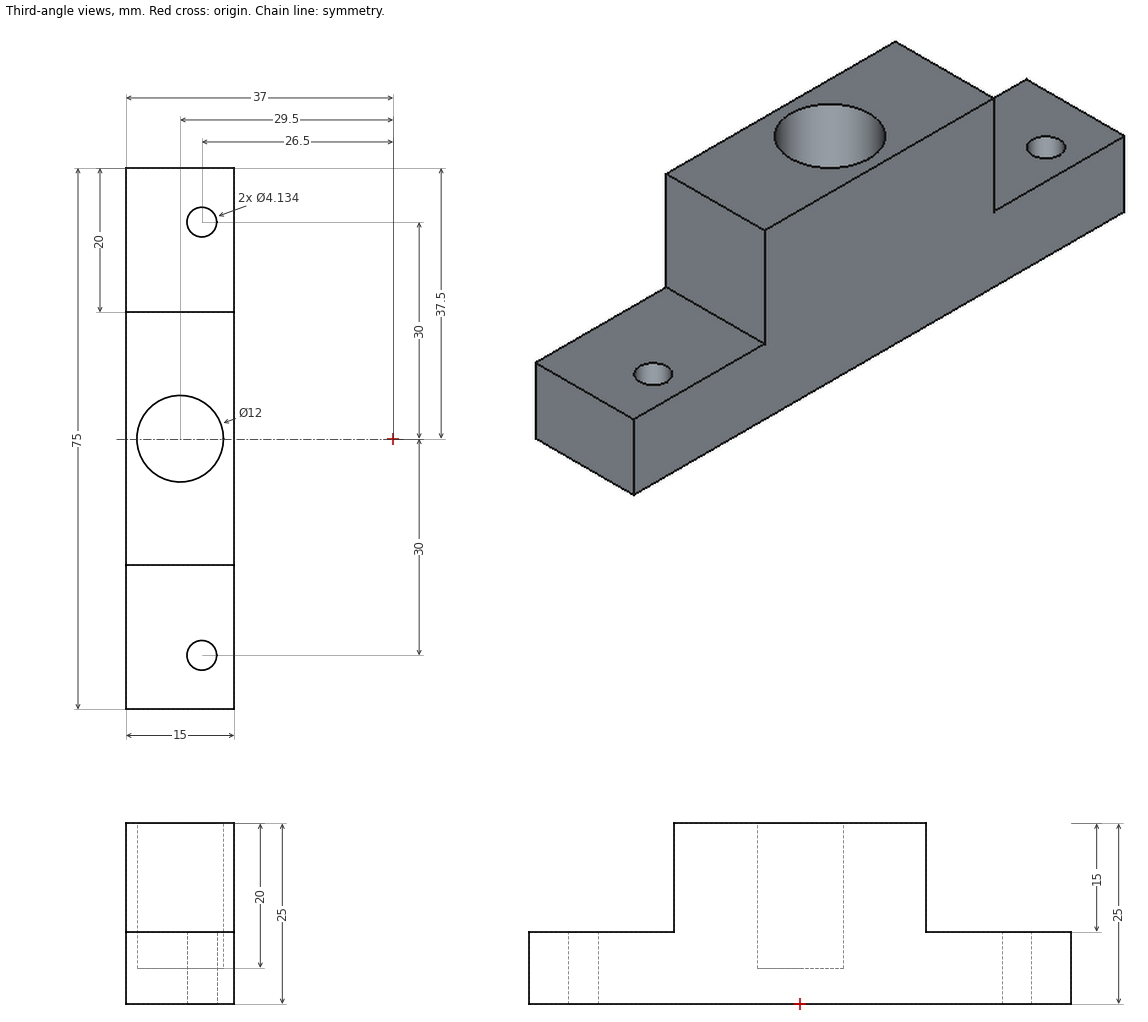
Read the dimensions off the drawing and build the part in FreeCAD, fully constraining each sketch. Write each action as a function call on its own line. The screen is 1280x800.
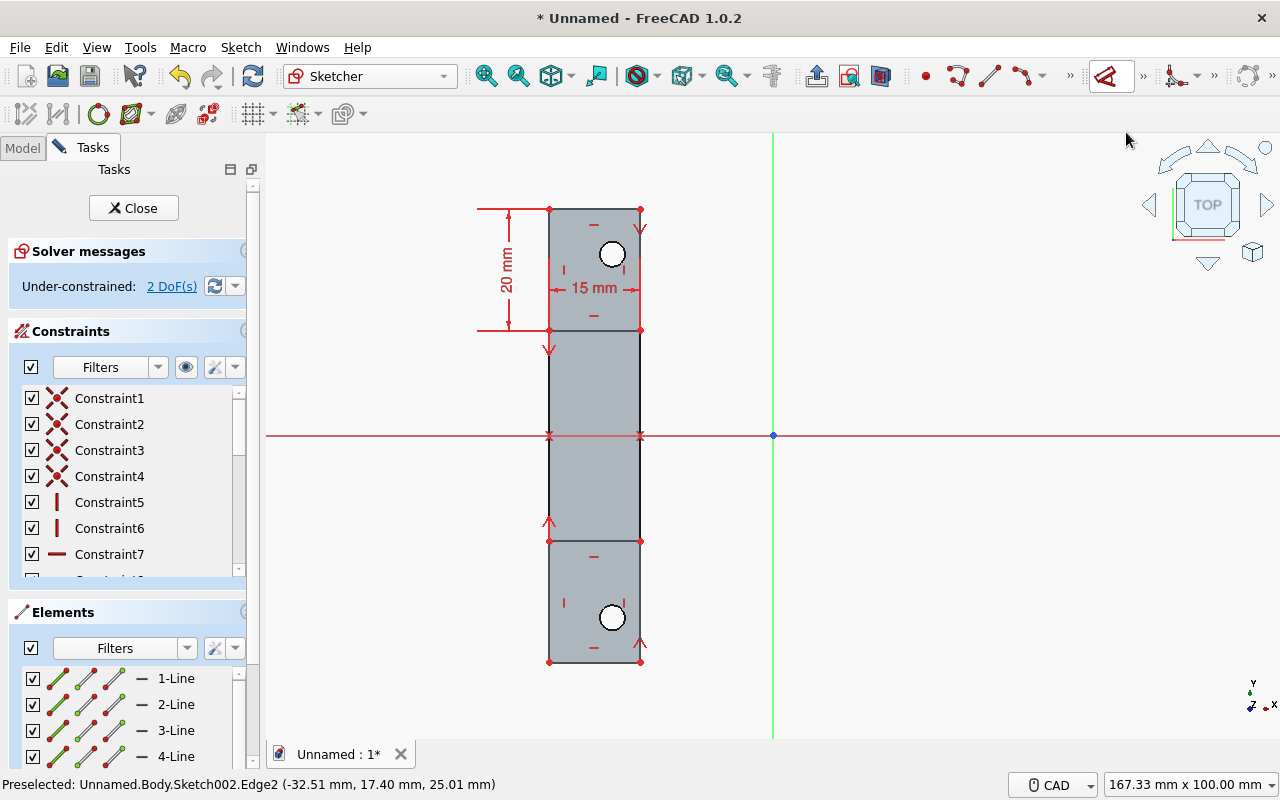
click(549, 209)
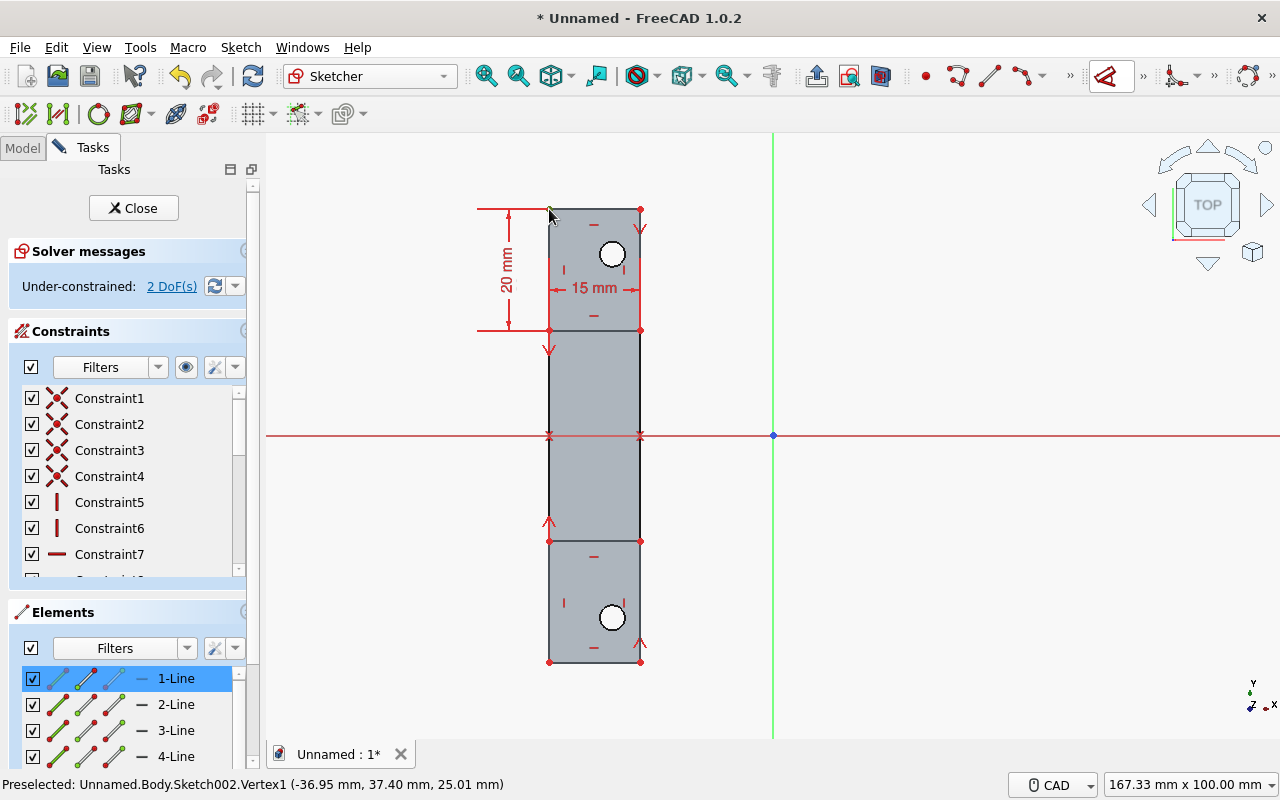
key(l)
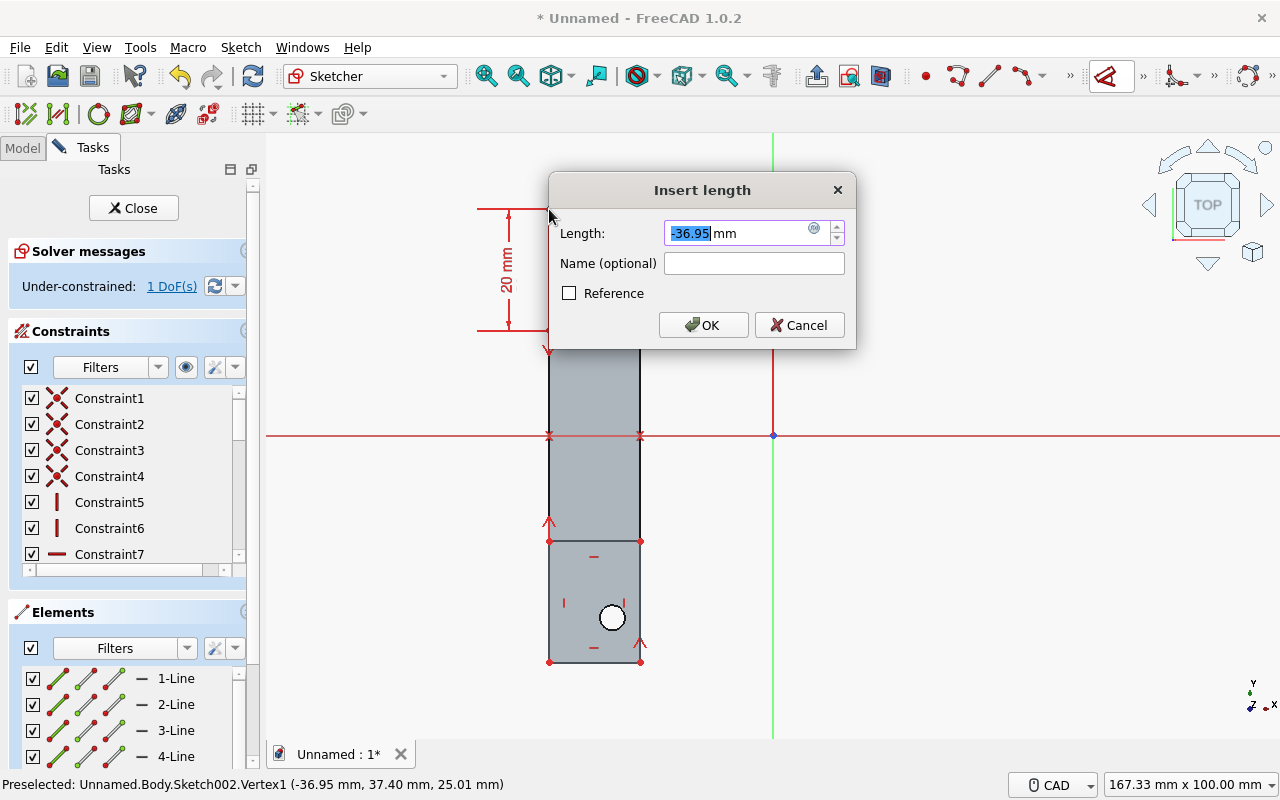
text(-37)
key(Return)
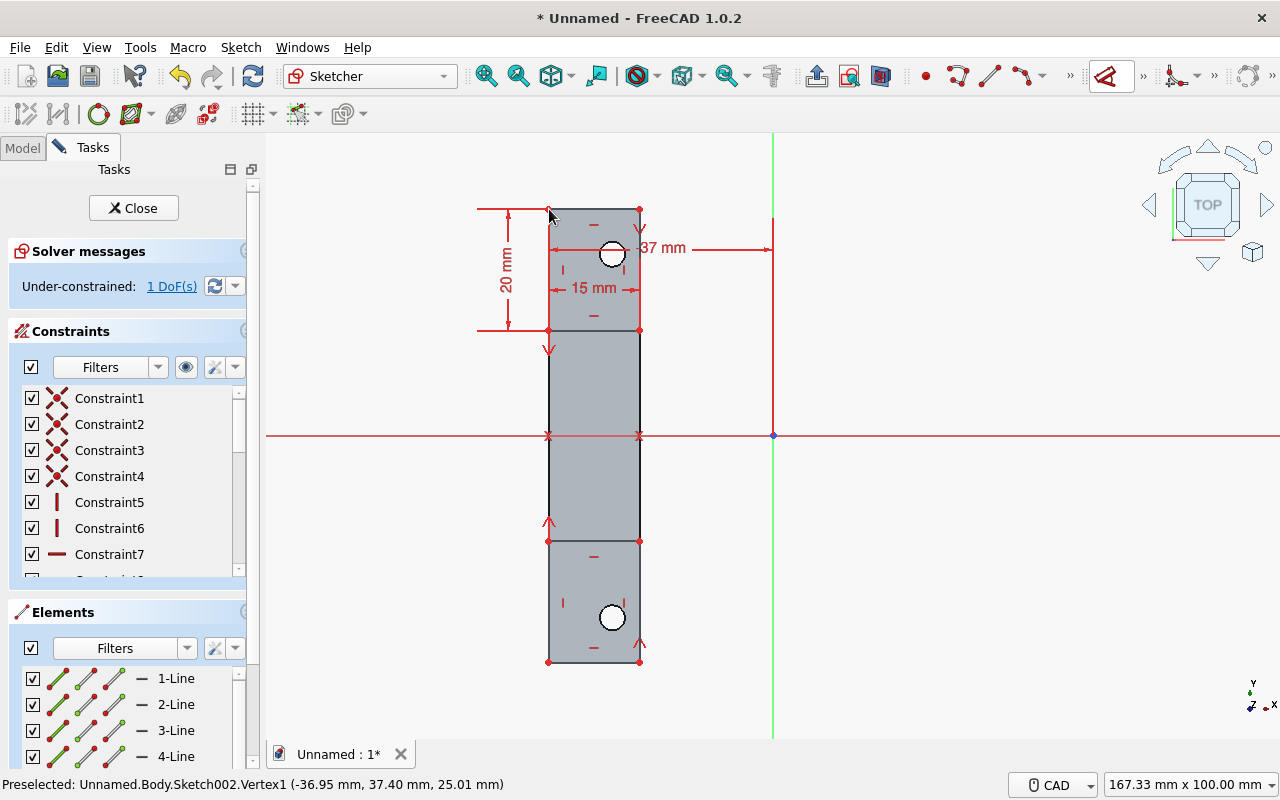
click(549, 209)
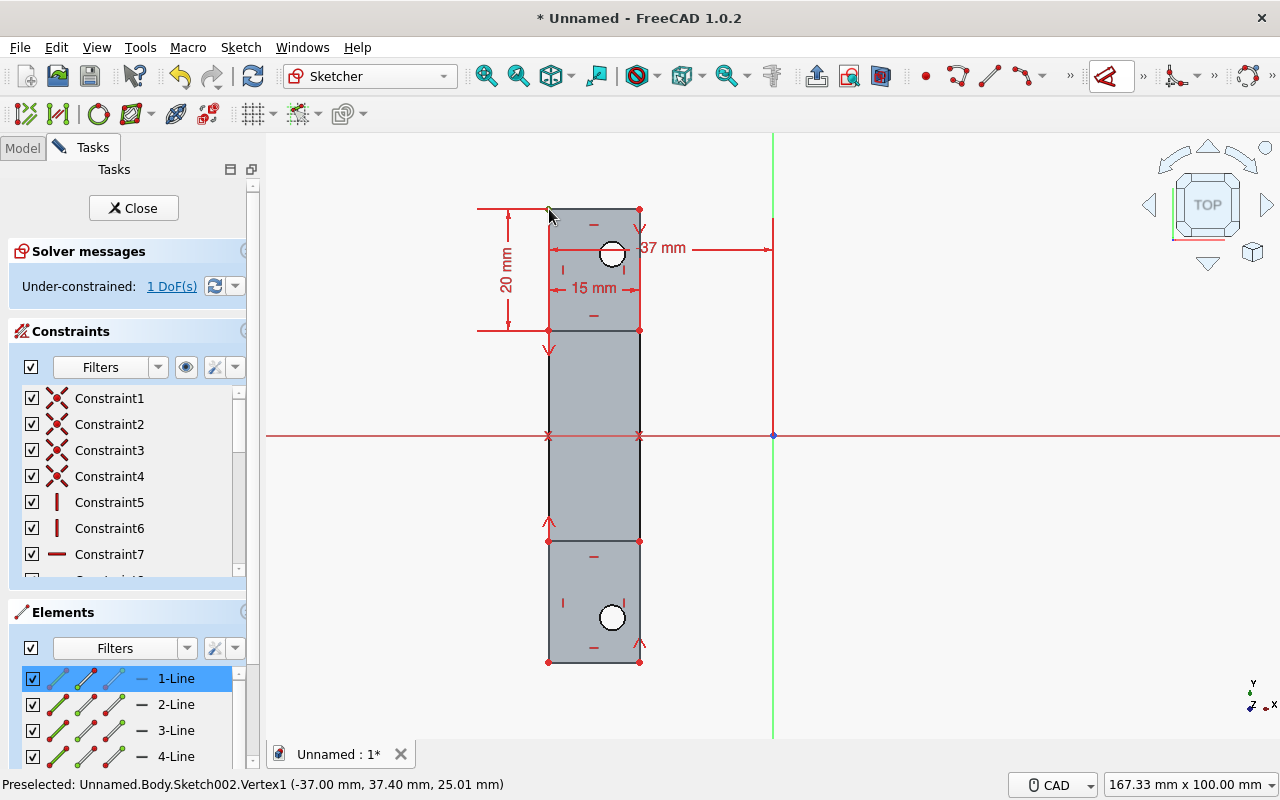
click(1128, 76)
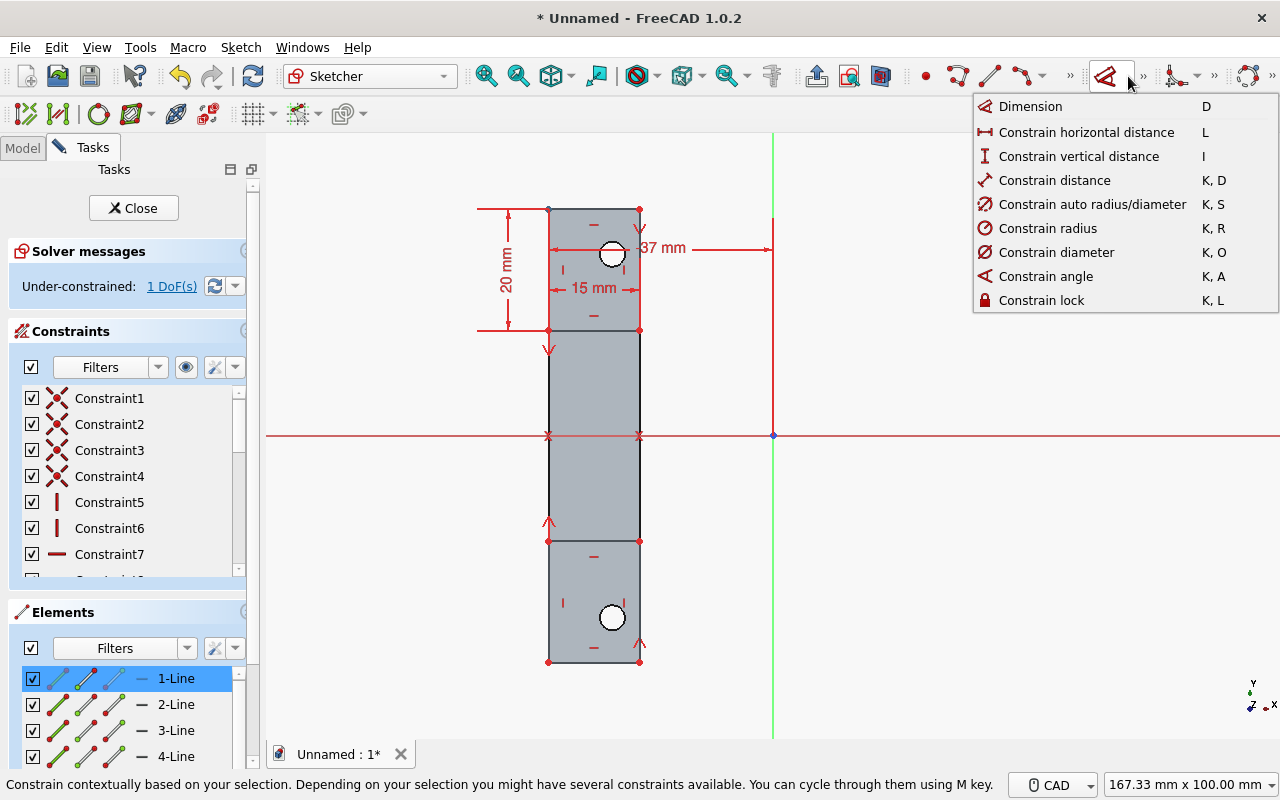
click(1126, 156)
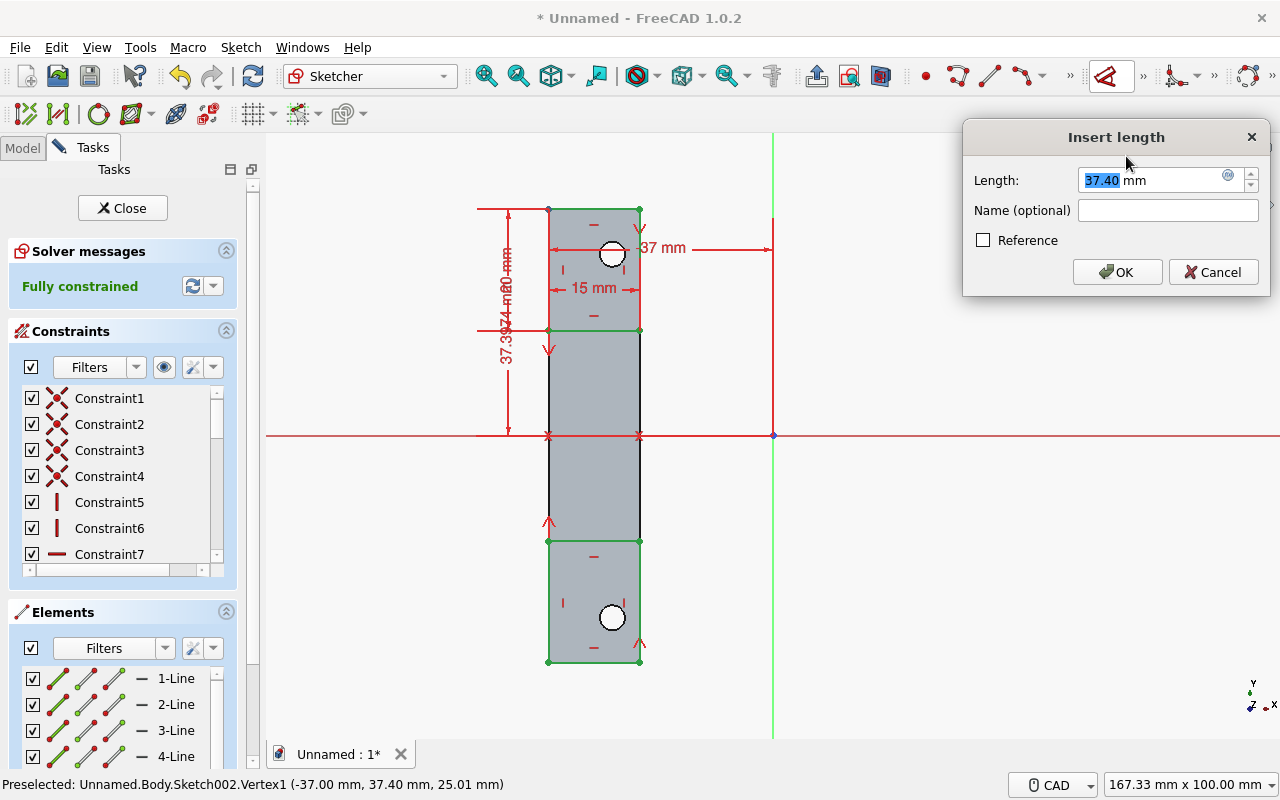
text(37.5)
key(Return)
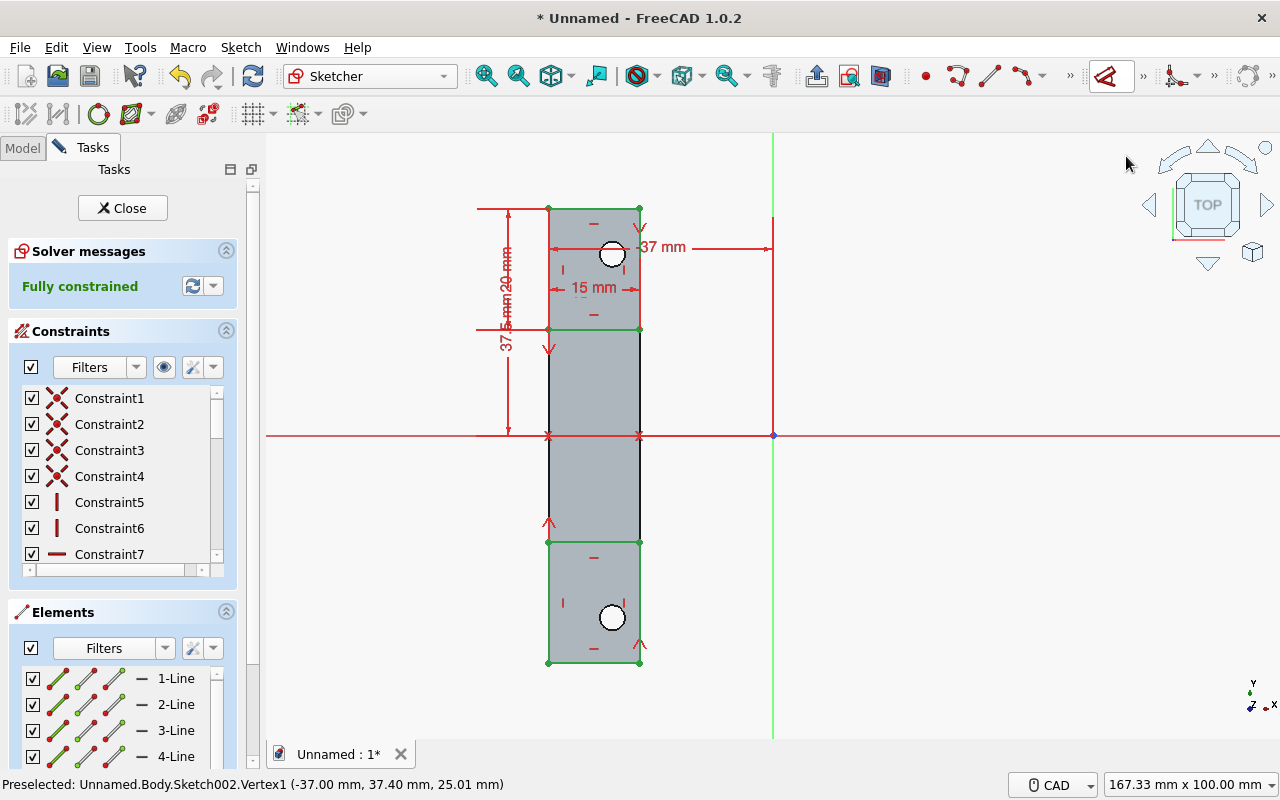
click(123, 208)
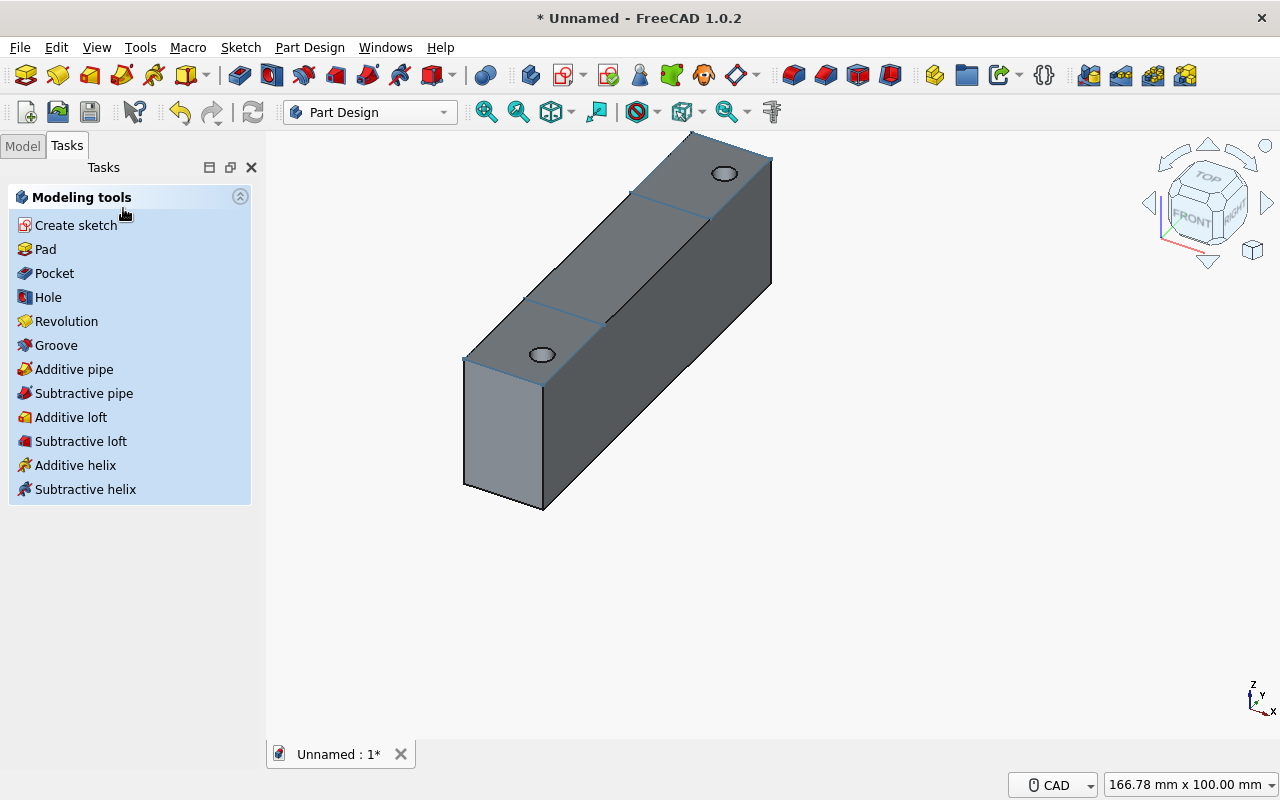
click(240, 76)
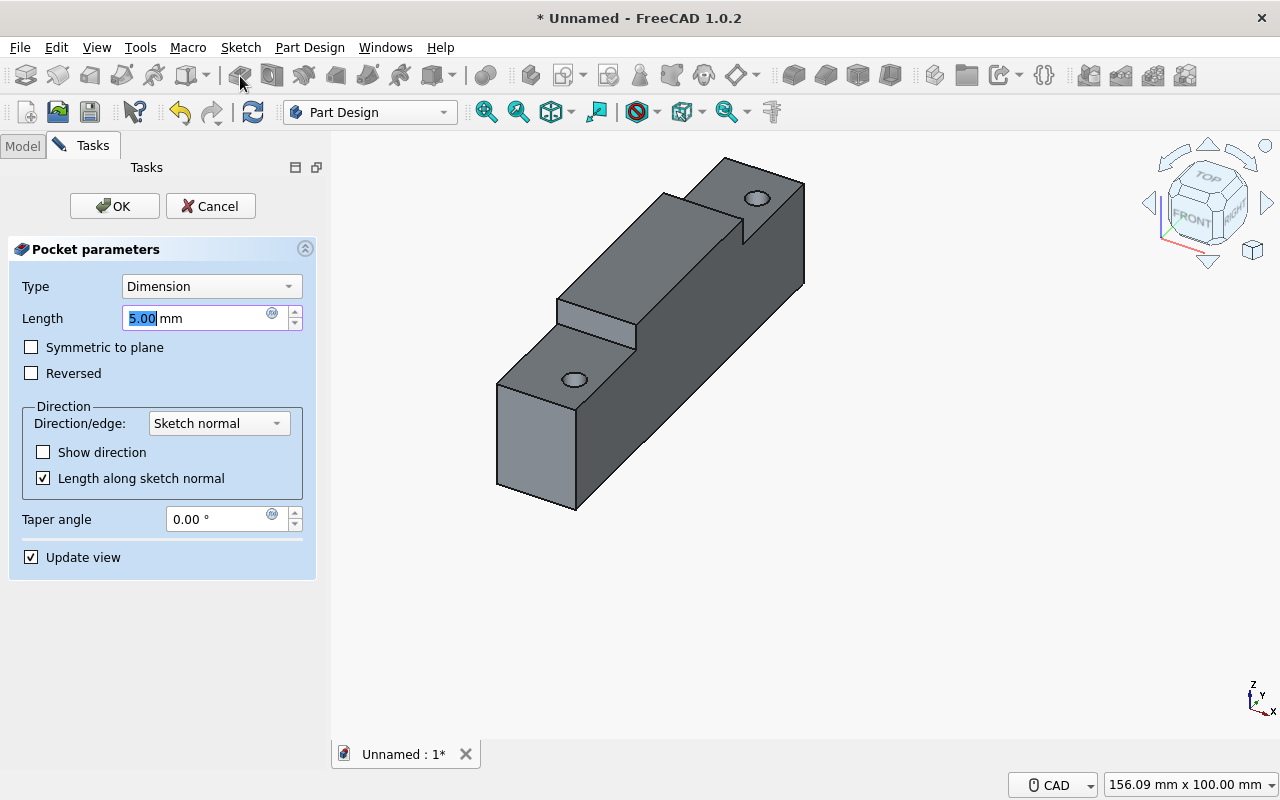
text(15)
key(Tab)